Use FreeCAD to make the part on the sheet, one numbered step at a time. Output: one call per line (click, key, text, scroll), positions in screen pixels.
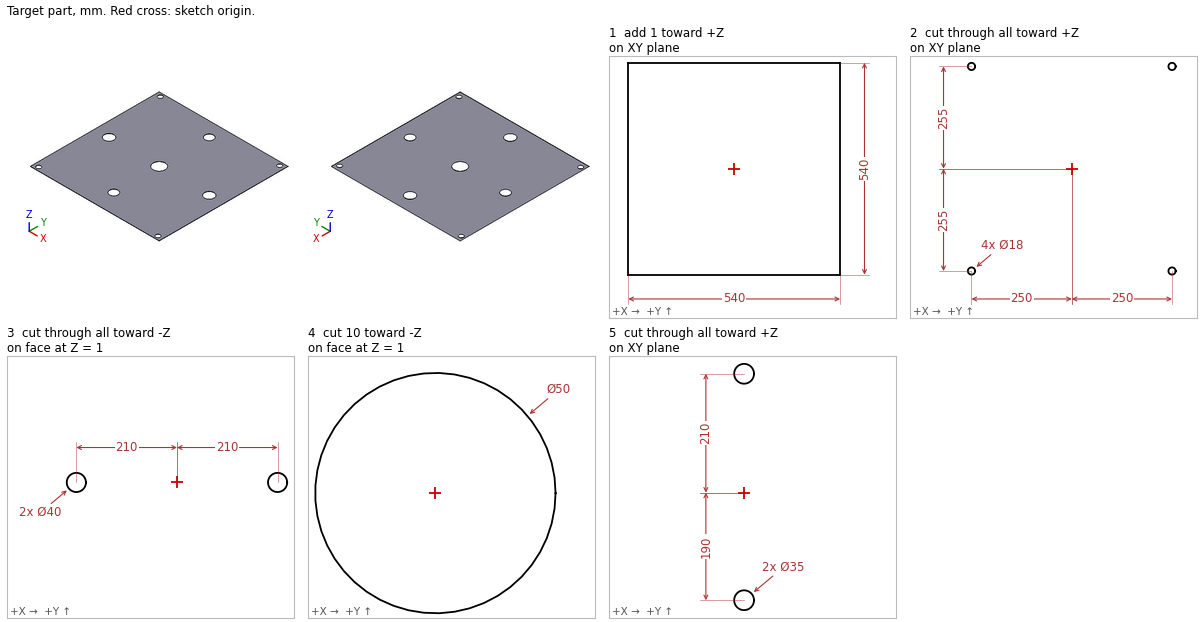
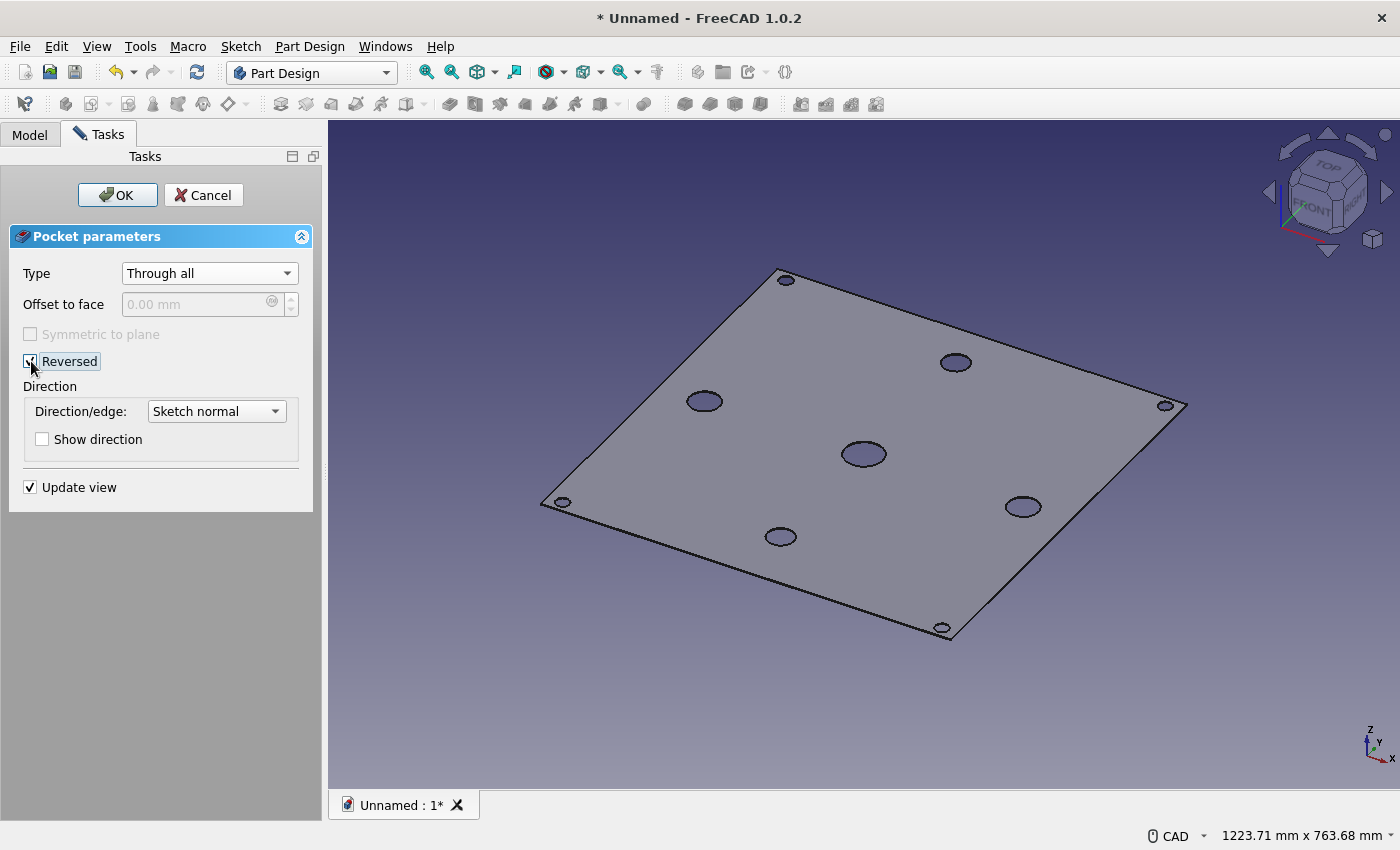
click(118, 195)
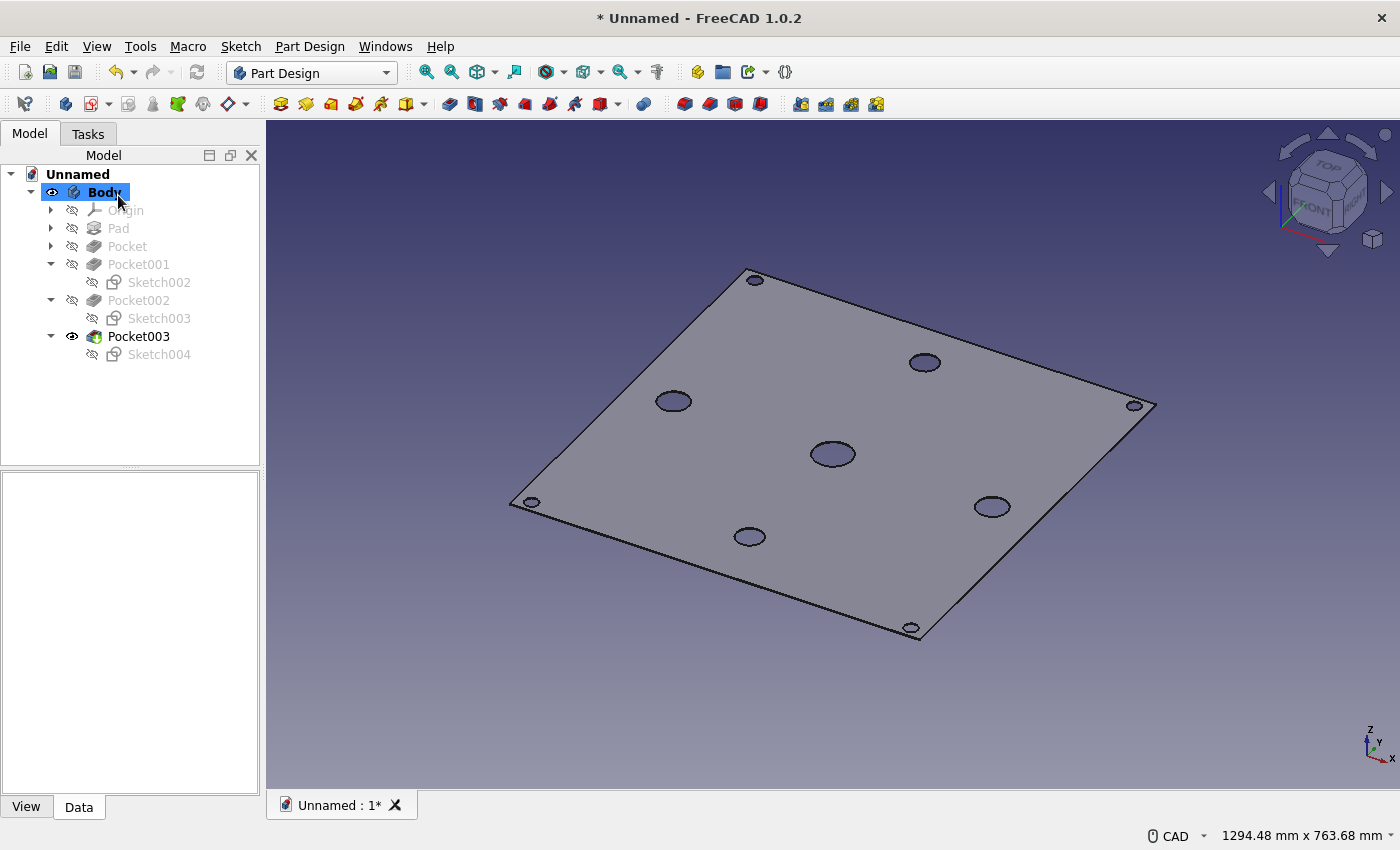
key(0)